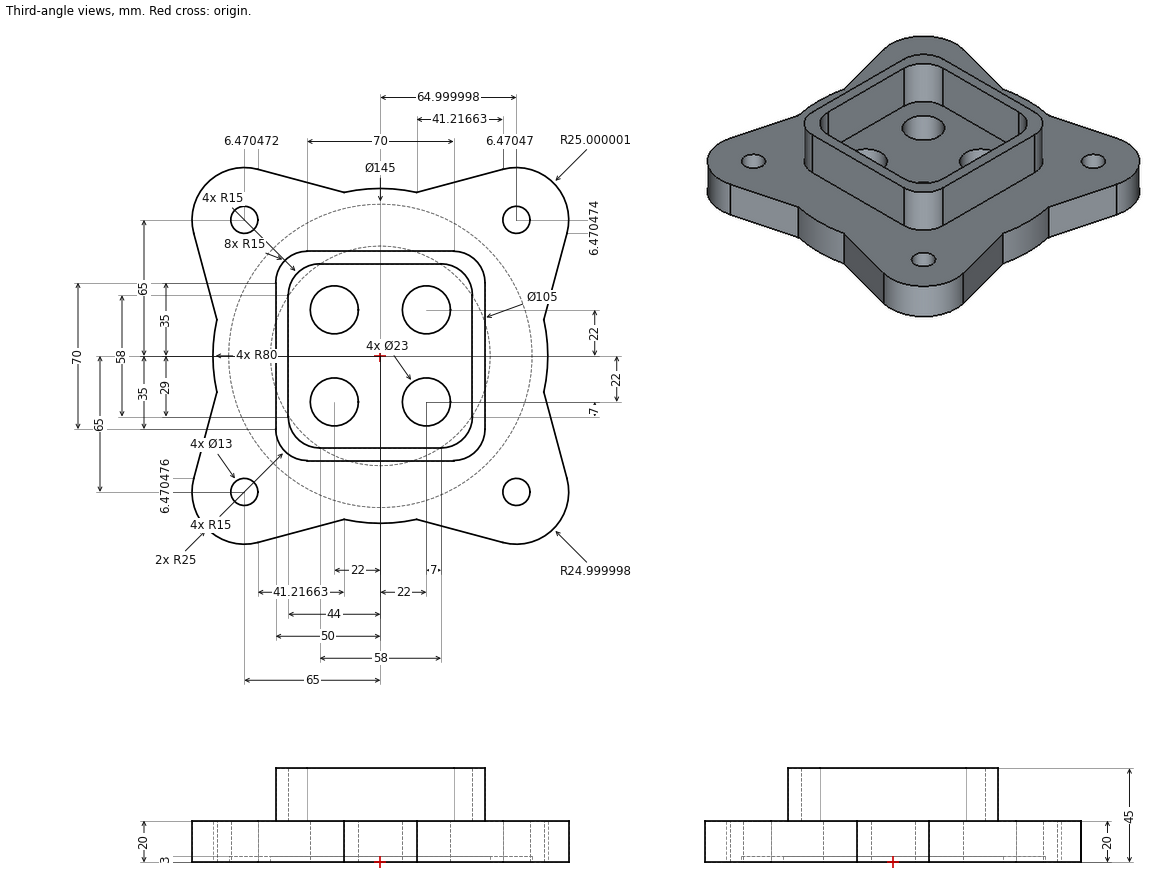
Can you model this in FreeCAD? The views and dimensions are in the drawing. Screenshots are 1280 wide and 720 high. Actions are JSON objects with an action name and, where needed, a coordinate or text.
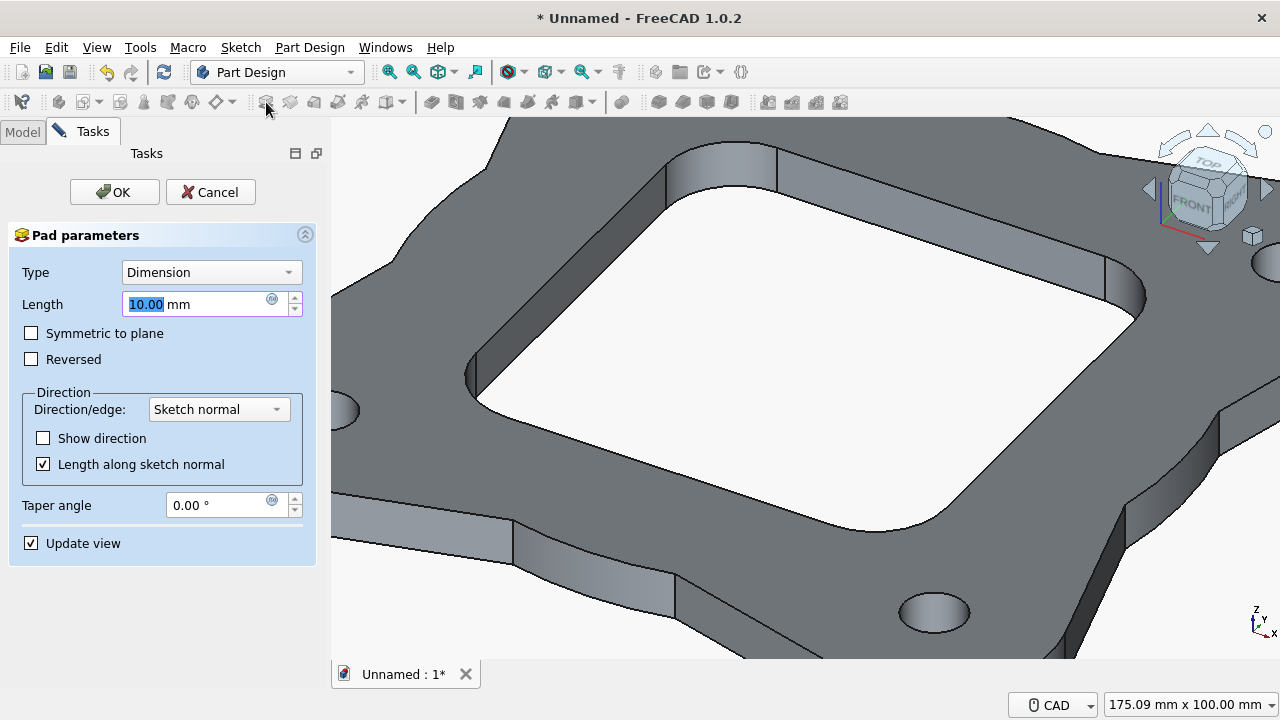
{"action": "type", "text": "20"}
{"action": "key", "text": "Tab"}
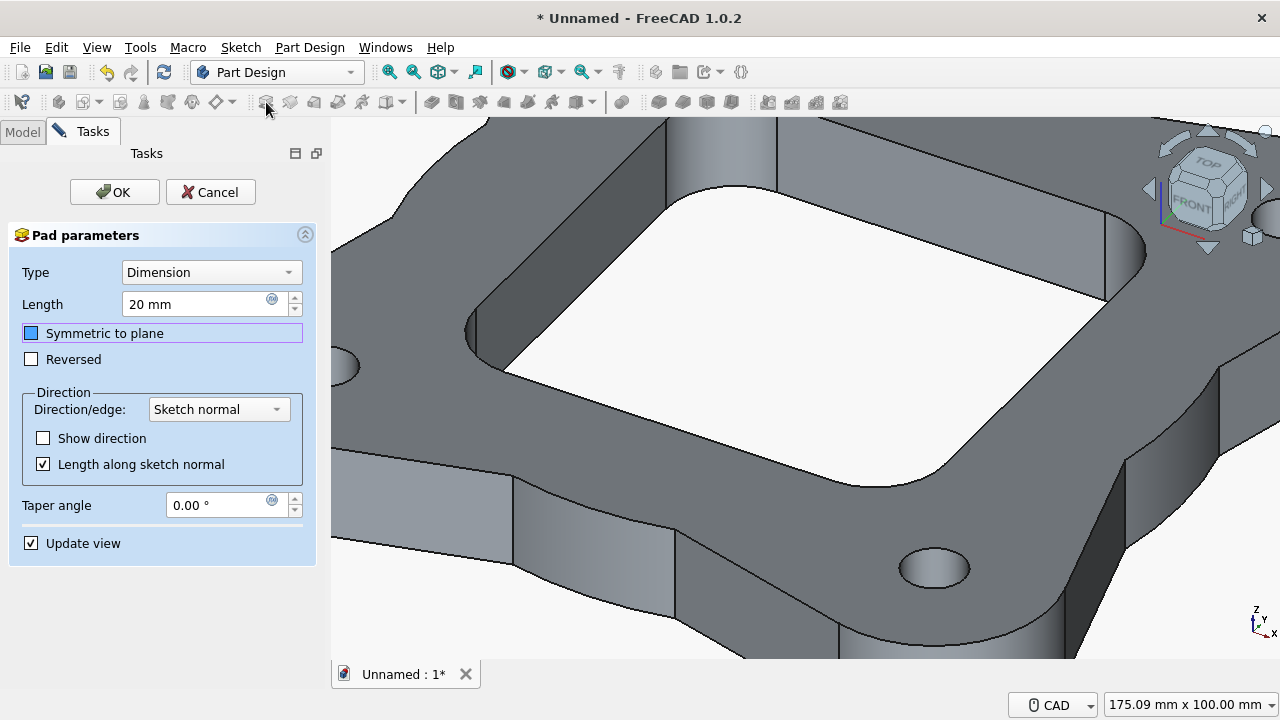
{"action": "left_click", "coordinate": [115, 192]}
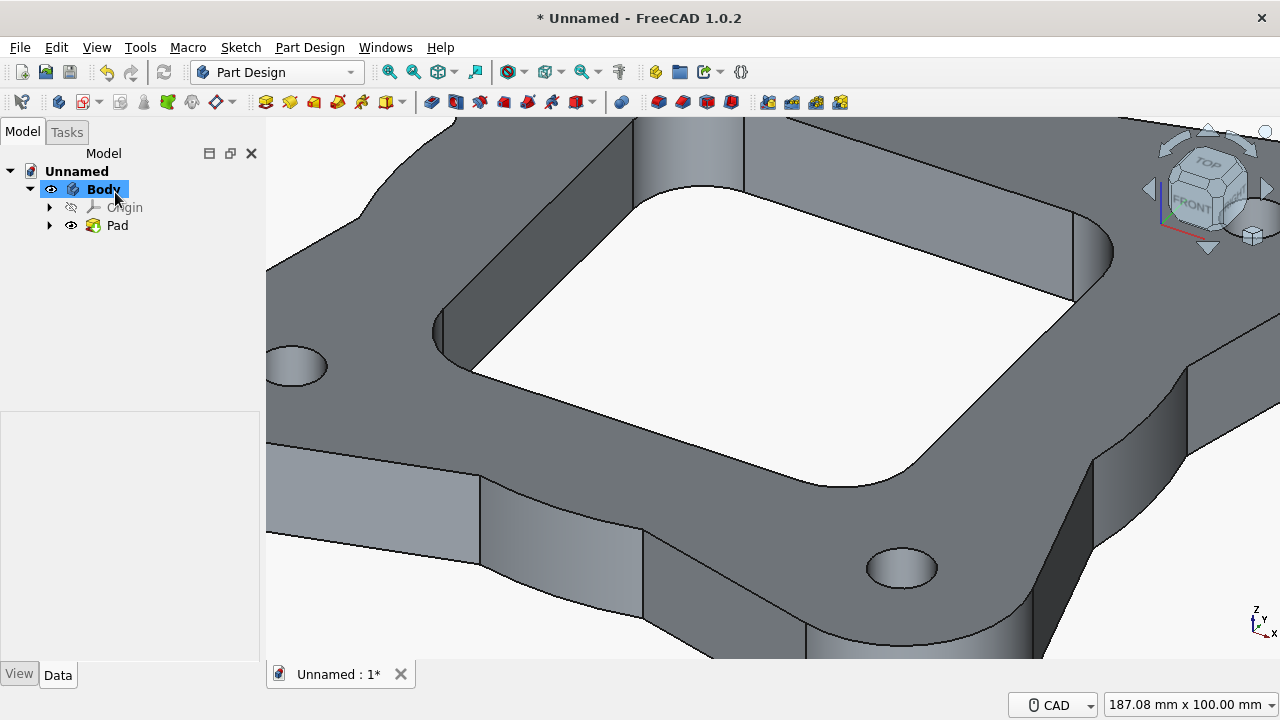
{"action": "left_click", "coordinate": [390, 72]}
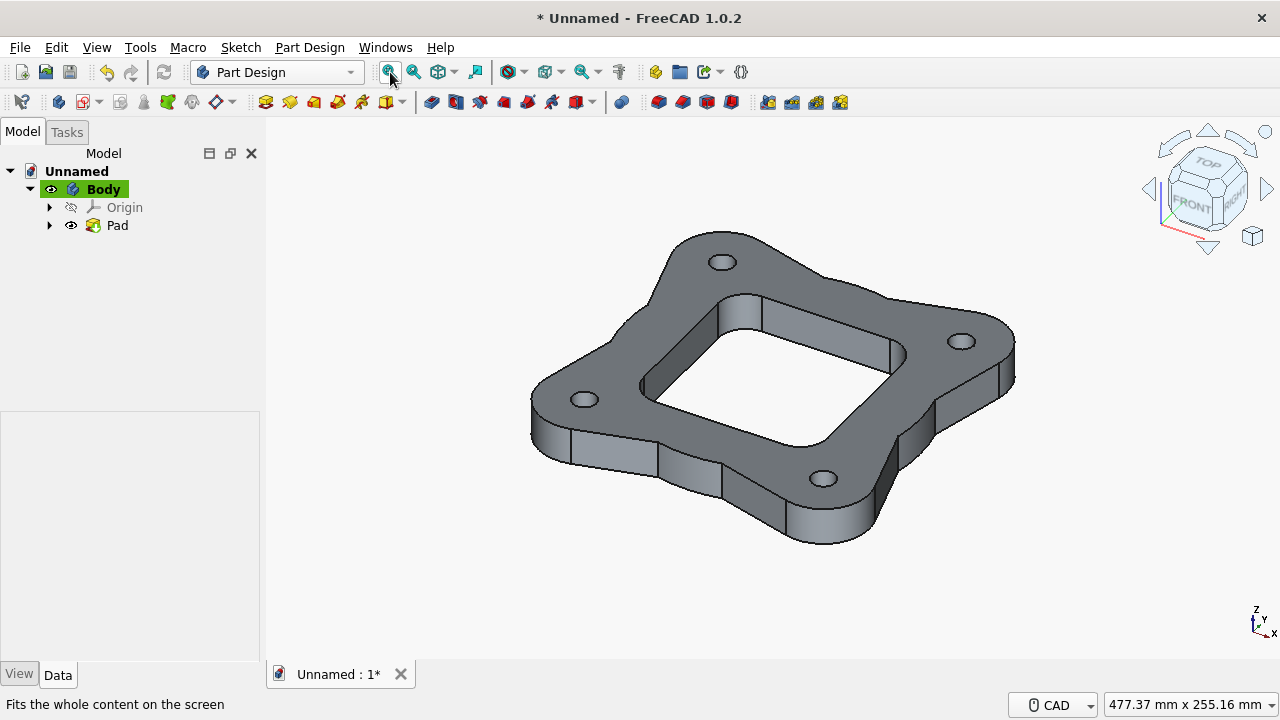
{"action": "left_click", "coordinate": [60, 102]}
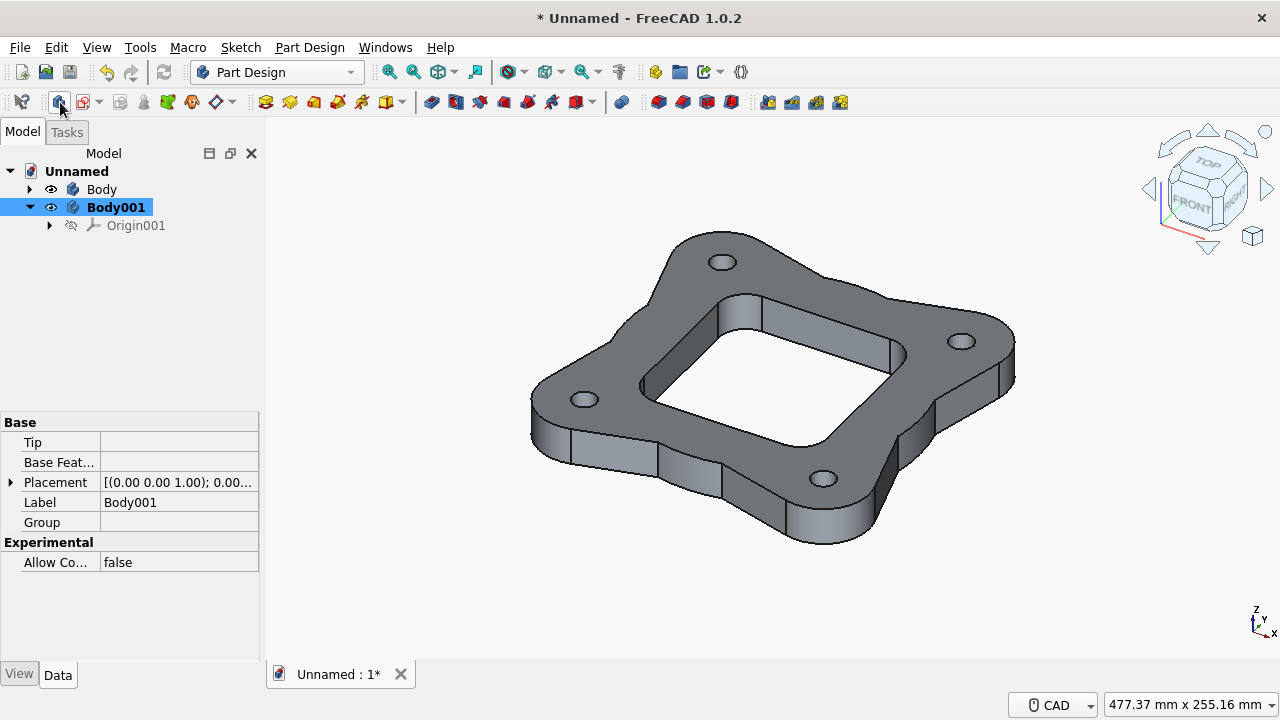
{"action": "left_click", "coordinate": [306, 619]}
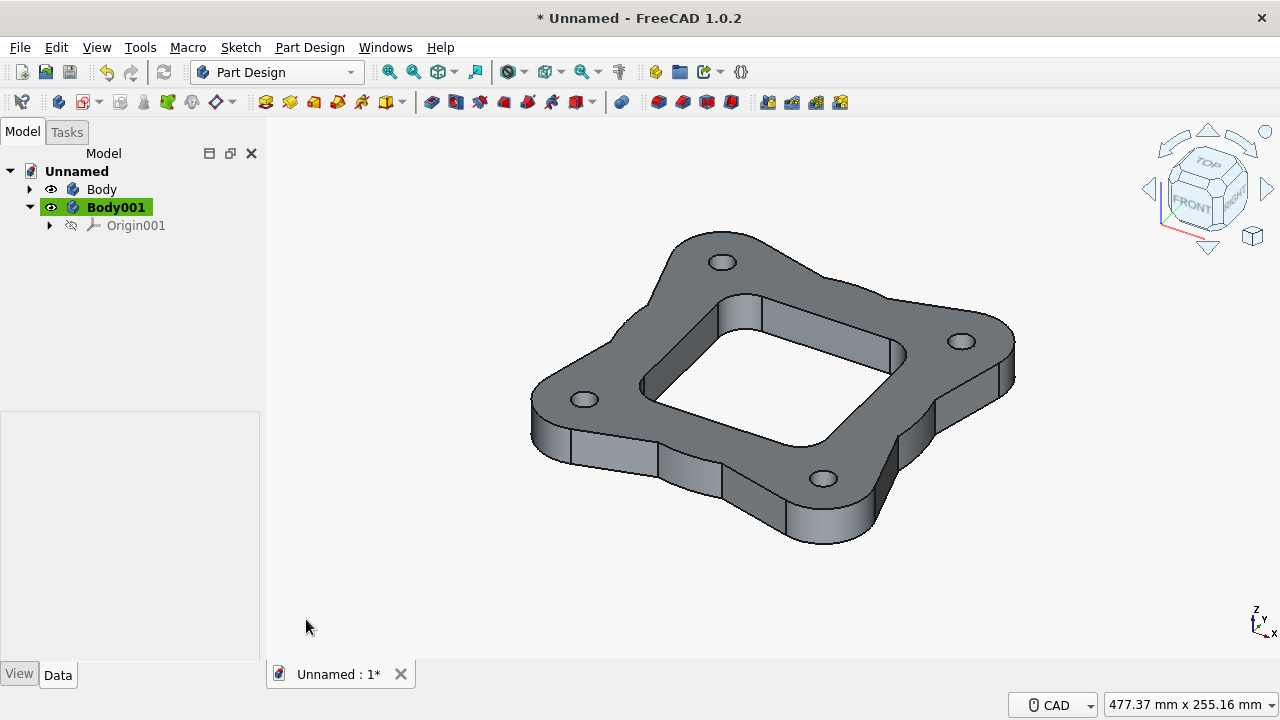
{"action": "left_click", "coordinate": [84, 102]}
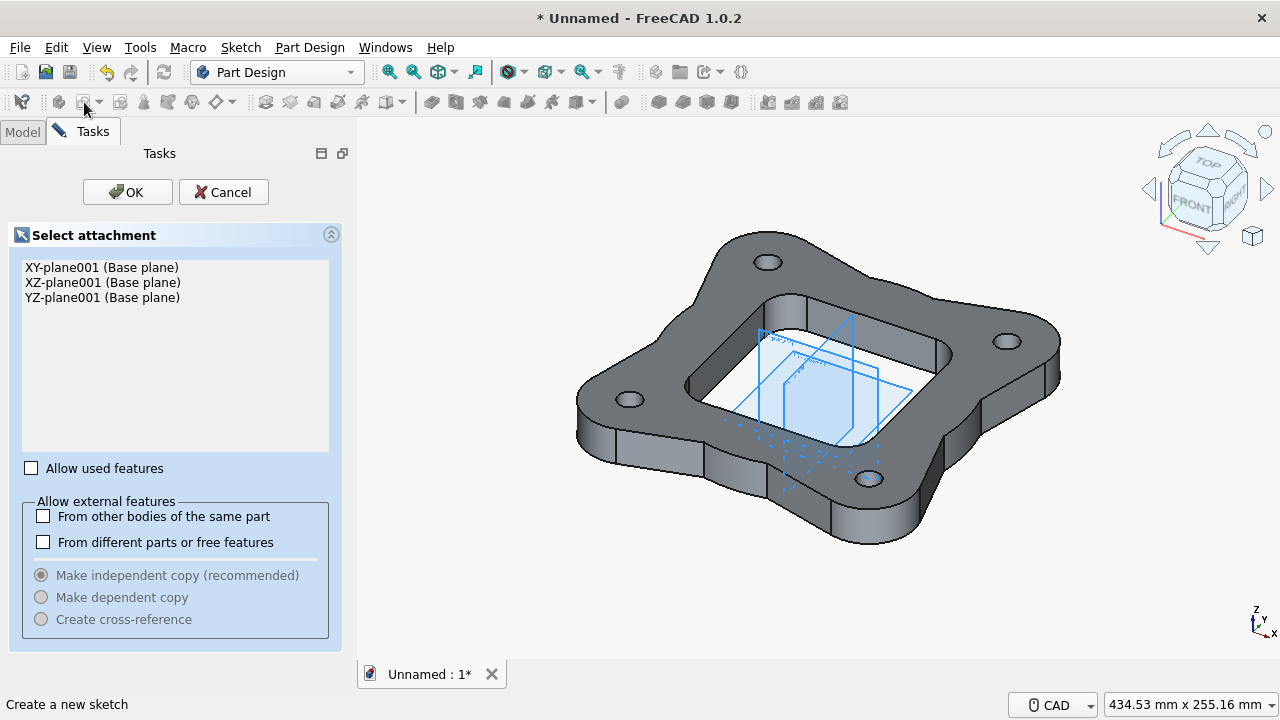
{"action": "left_click", "coordinate": [82, 268]}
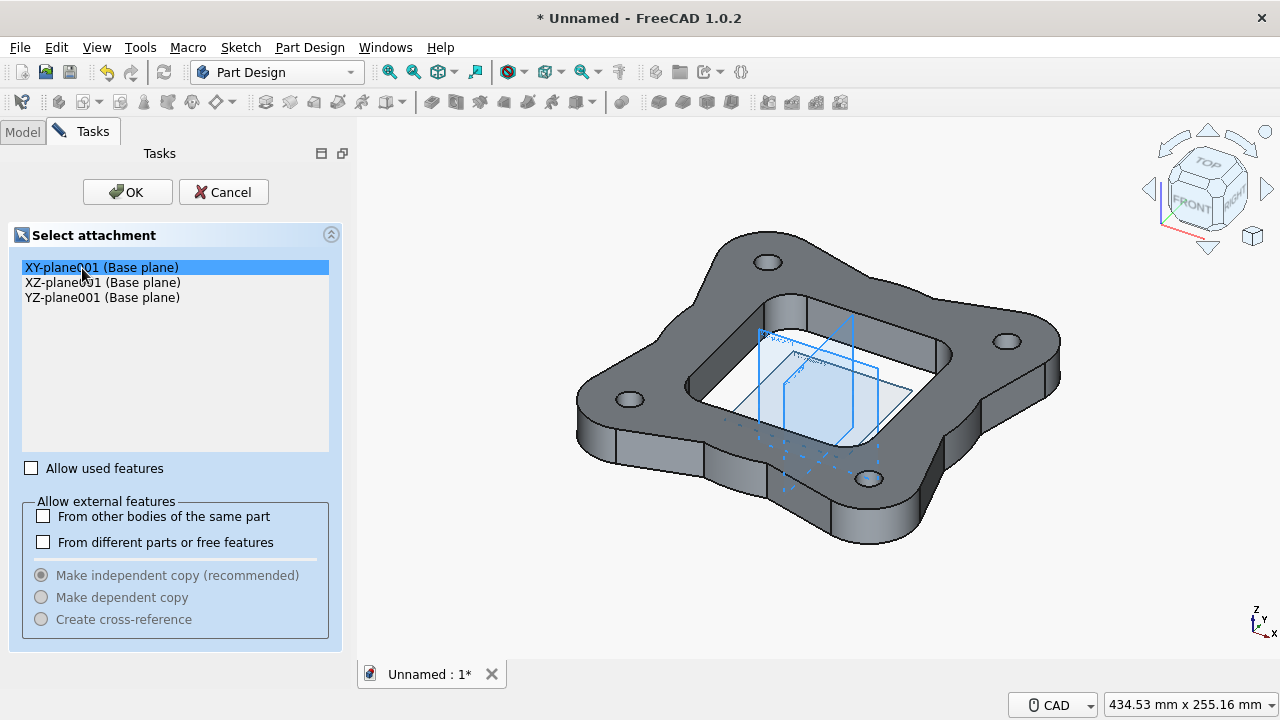
{"action": "left_click", "coordinate": [128, 192]}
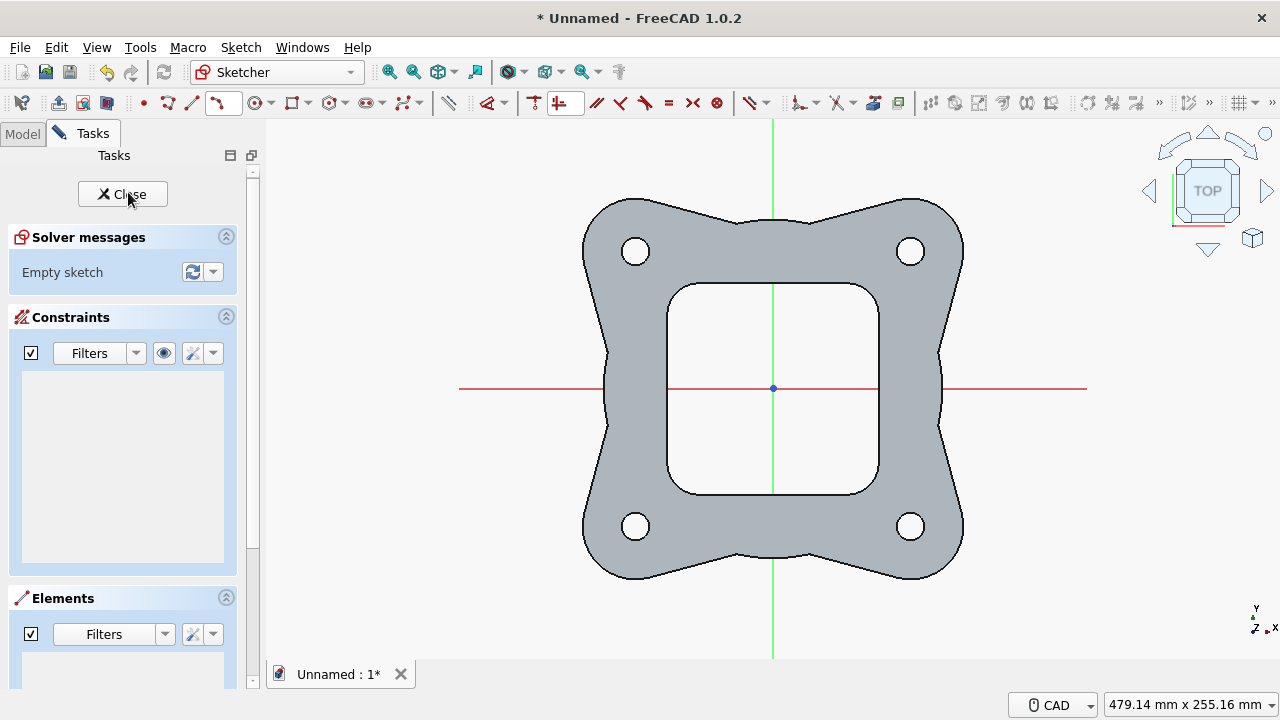
{"action": "scroll", "coordinate": [856, 389], "scroll_direction": "up", "scroll_amount": 3}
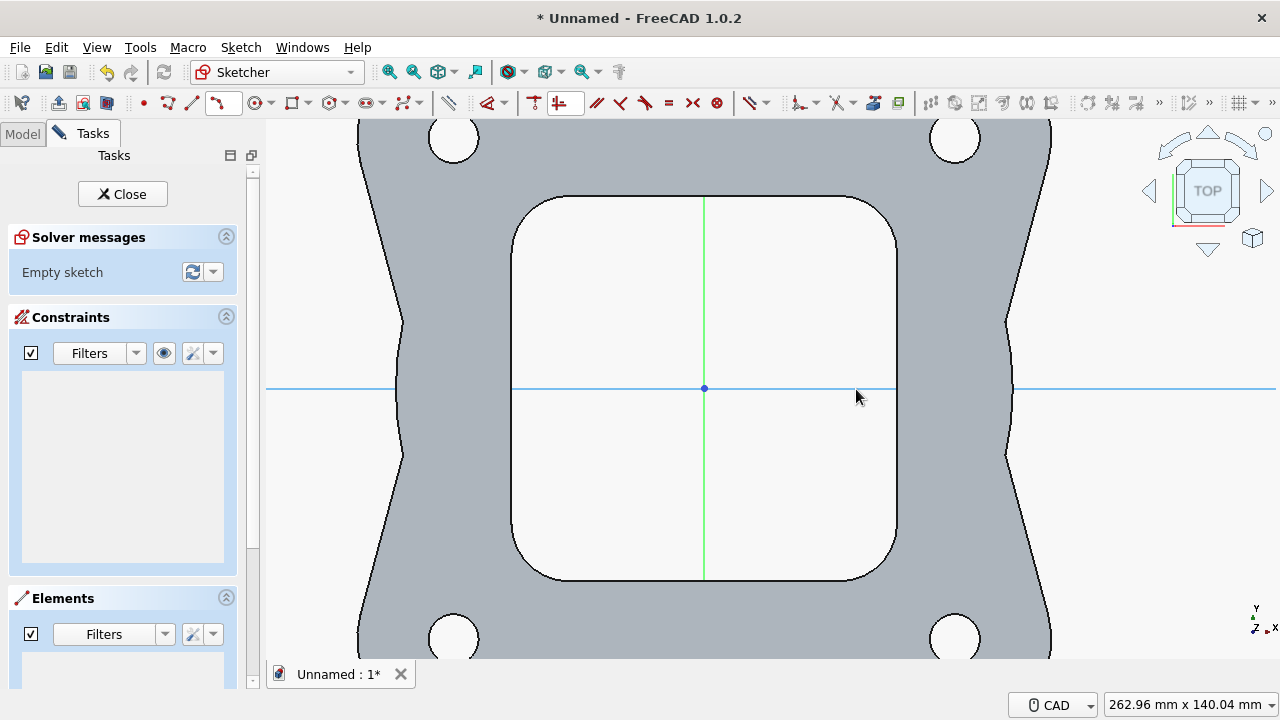
{"action": "key", "text": "g l"}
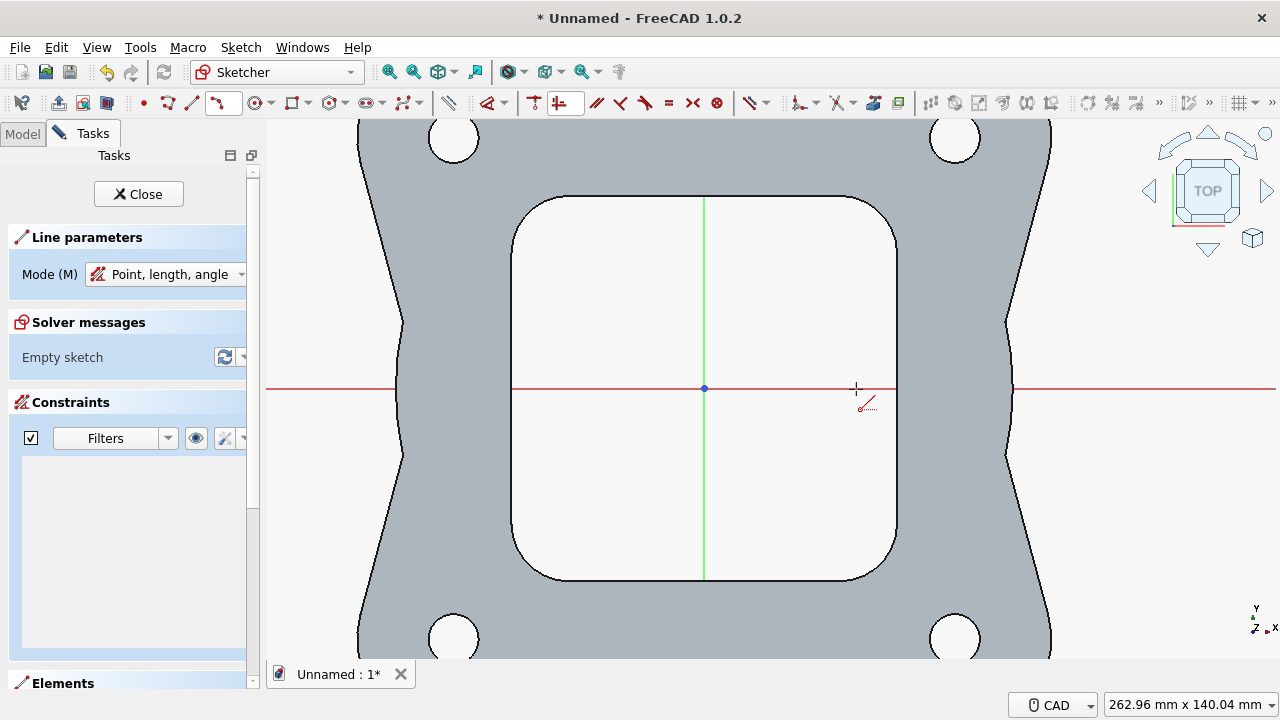
{"action": "left_click", "coordinate": [535, 277]}
{"action": "left_click", "coordinate": [535, 500]}